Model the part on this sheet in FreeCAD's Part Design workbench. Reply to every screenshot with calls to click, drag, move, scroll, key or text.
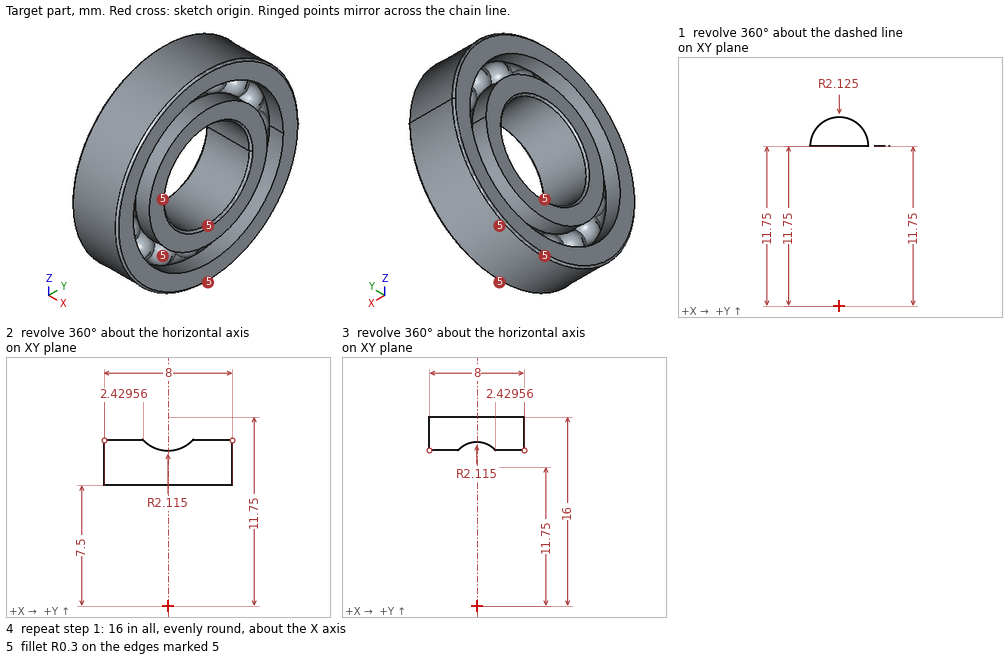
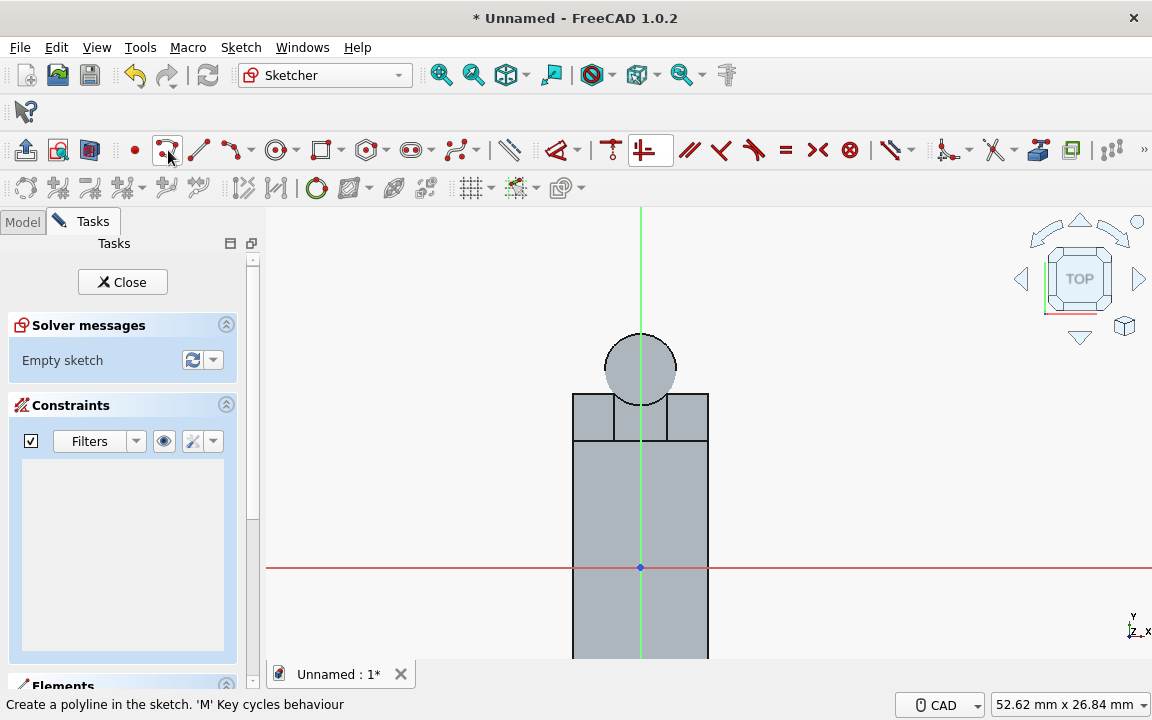
click(667, 346)
click(708, 346)
click(708, 298)
click(573, 298)
click(573, 346)
click(614, 346)
right_click(614, 346)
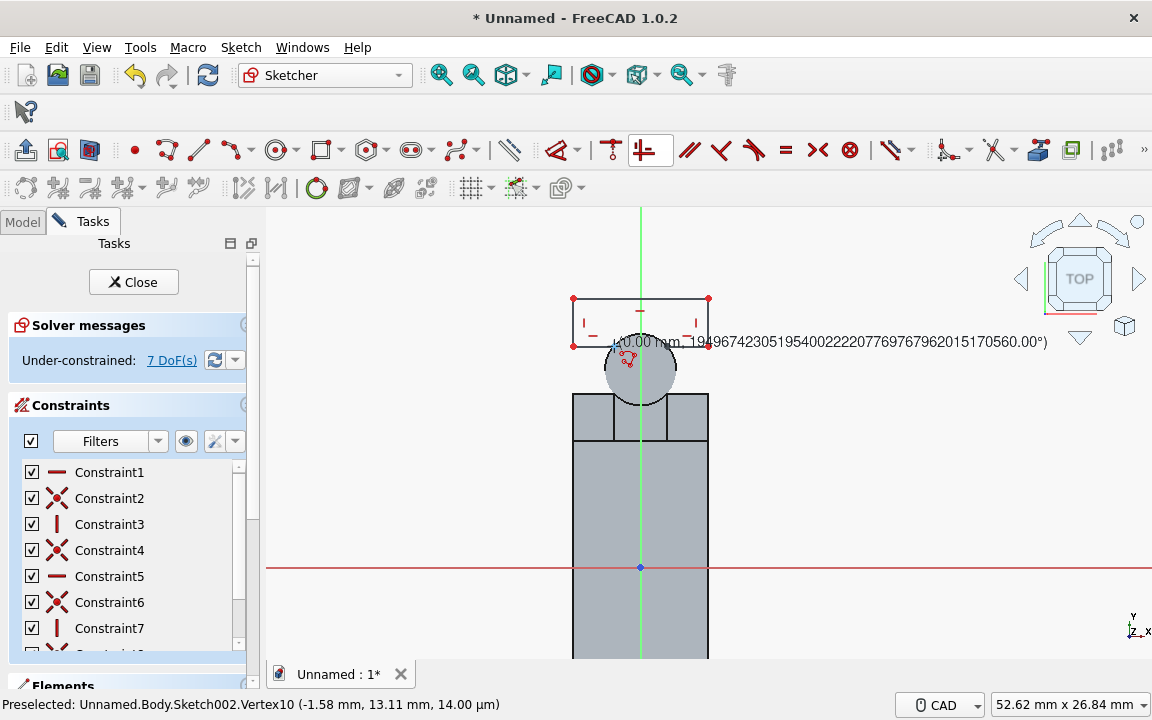
click(232, 150)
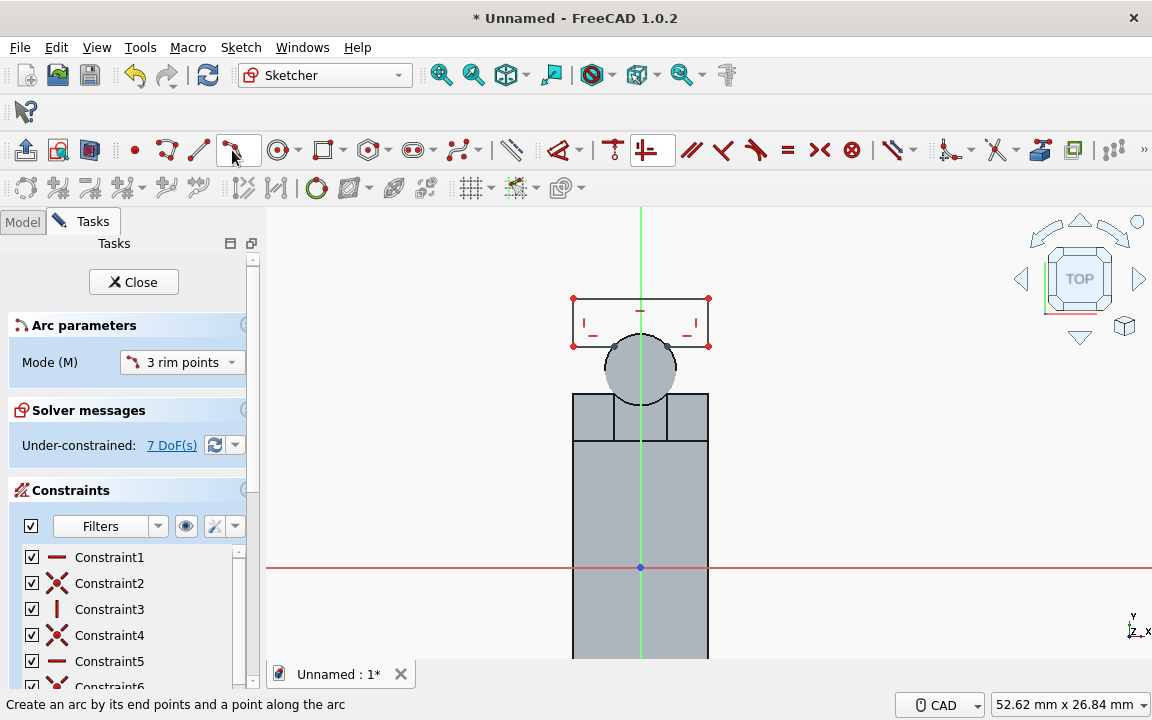
click(614, 347)
click(667, 347)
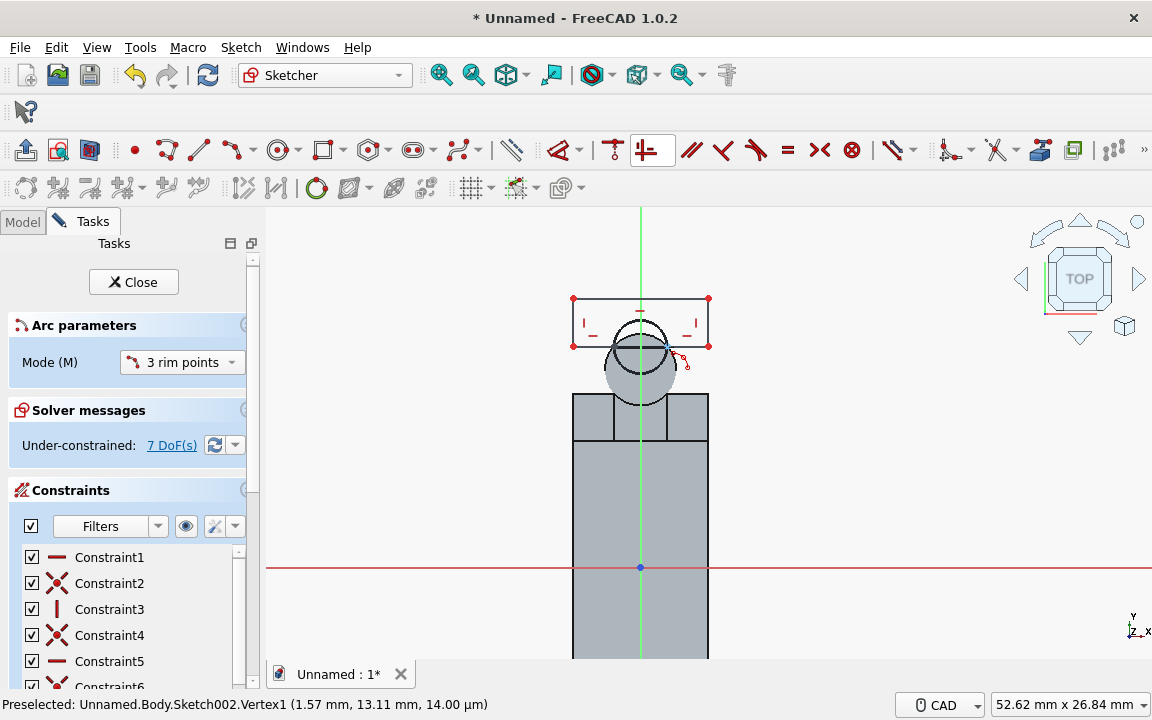
scroll(652, 336, up, 3)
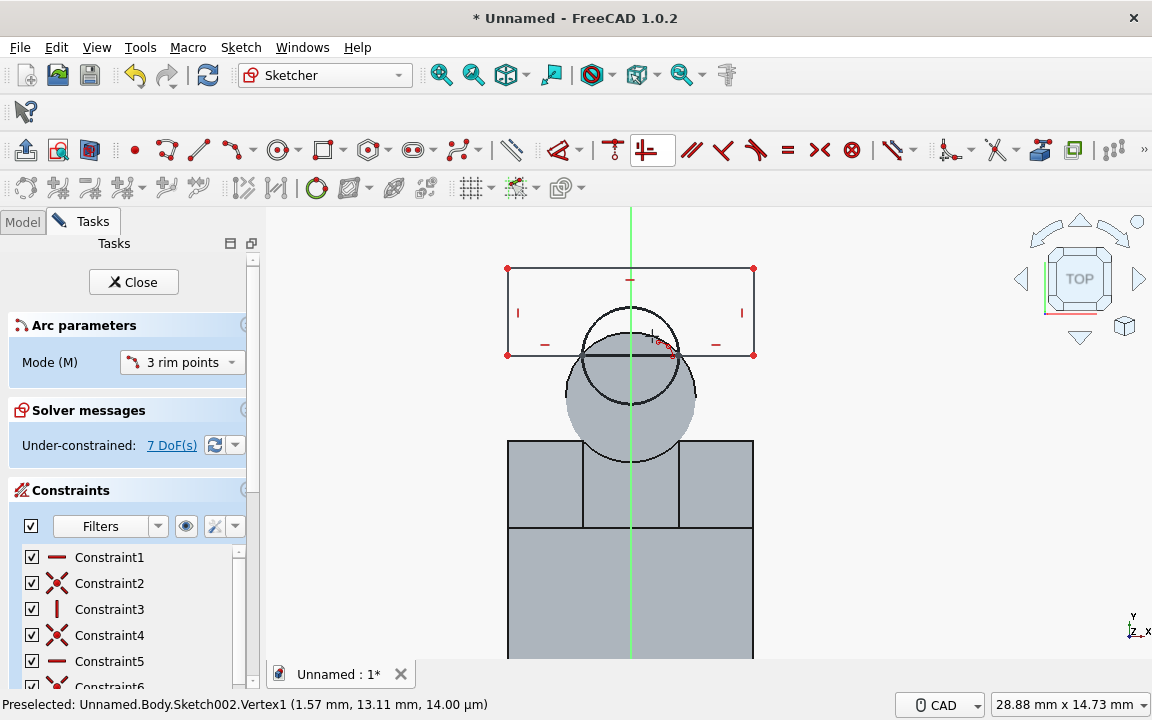
click(652, 336)
key(Escape)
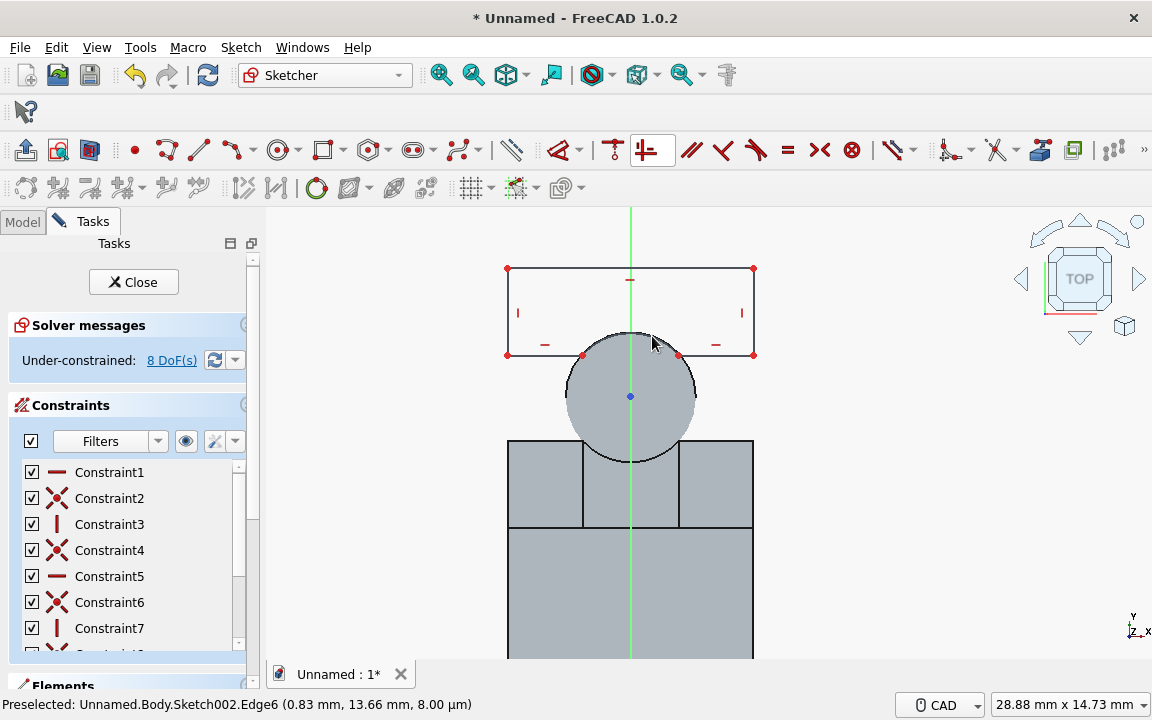
click(631, 396)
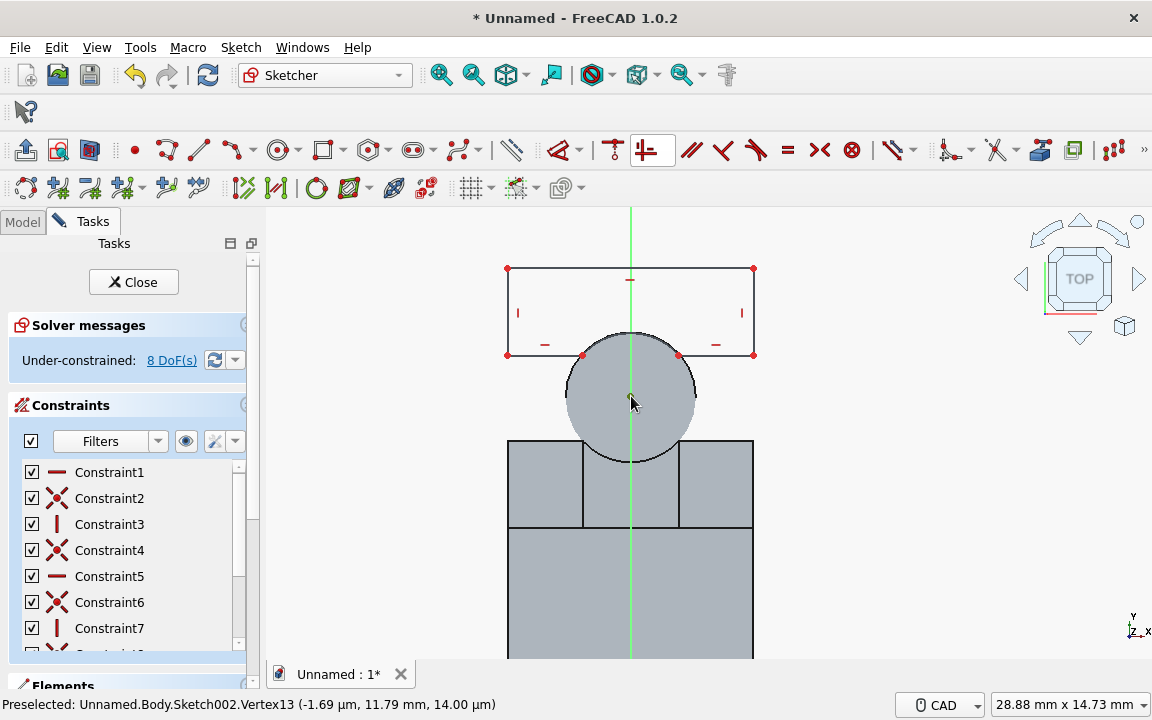
click(631, 603)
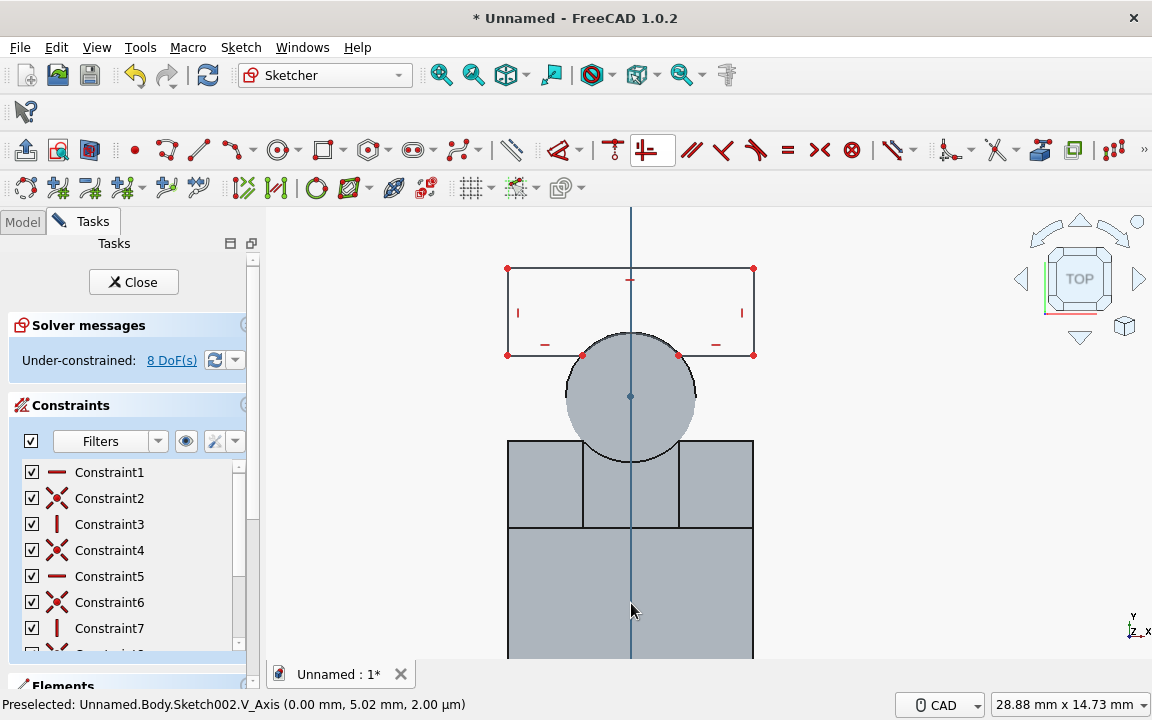
click(614, 150)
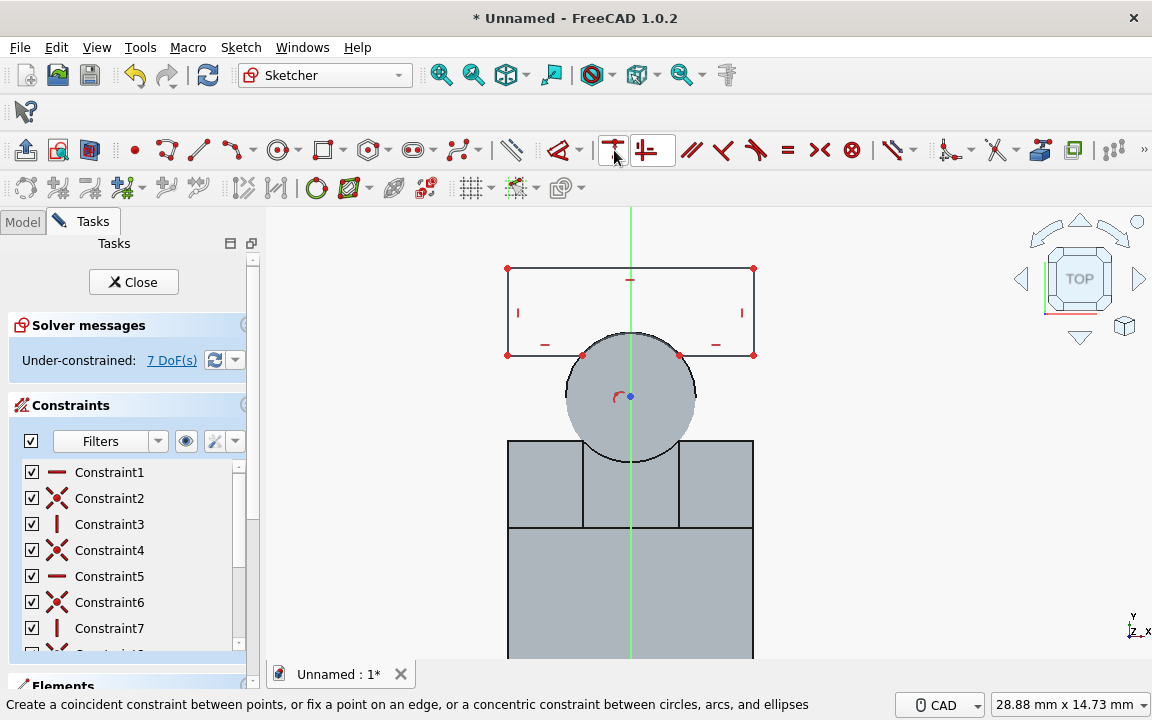
click(754, 356)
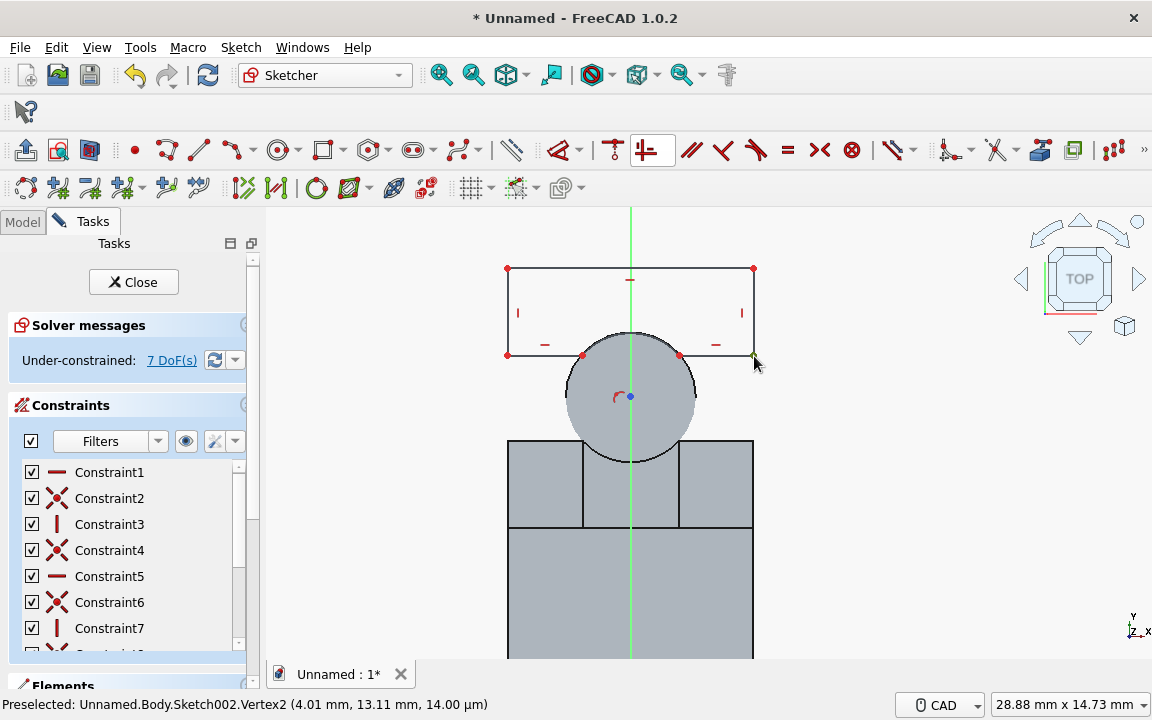
click(508, 356)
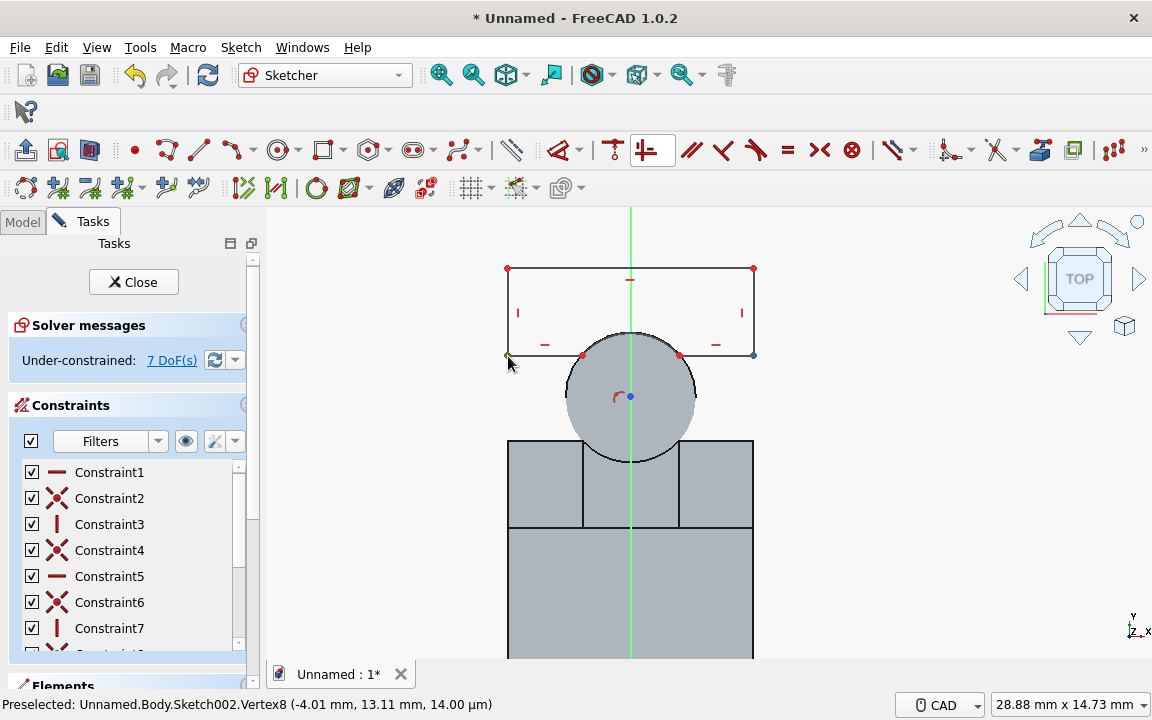
click(631, 603)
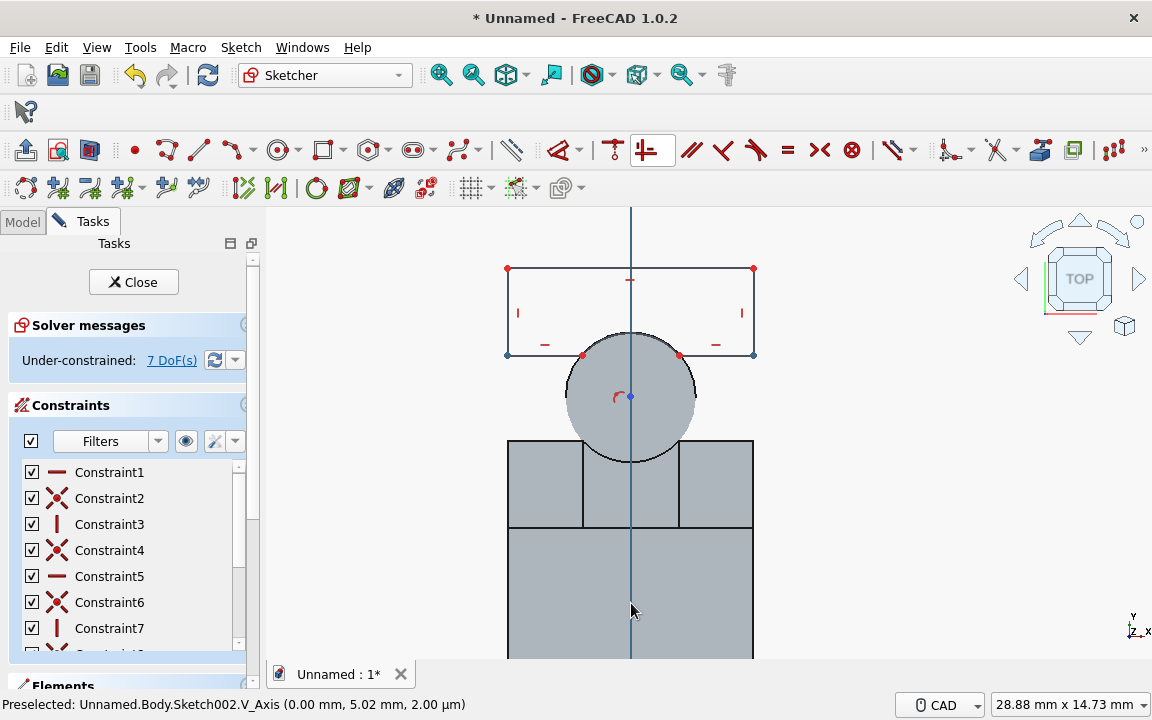
click(820, 150)